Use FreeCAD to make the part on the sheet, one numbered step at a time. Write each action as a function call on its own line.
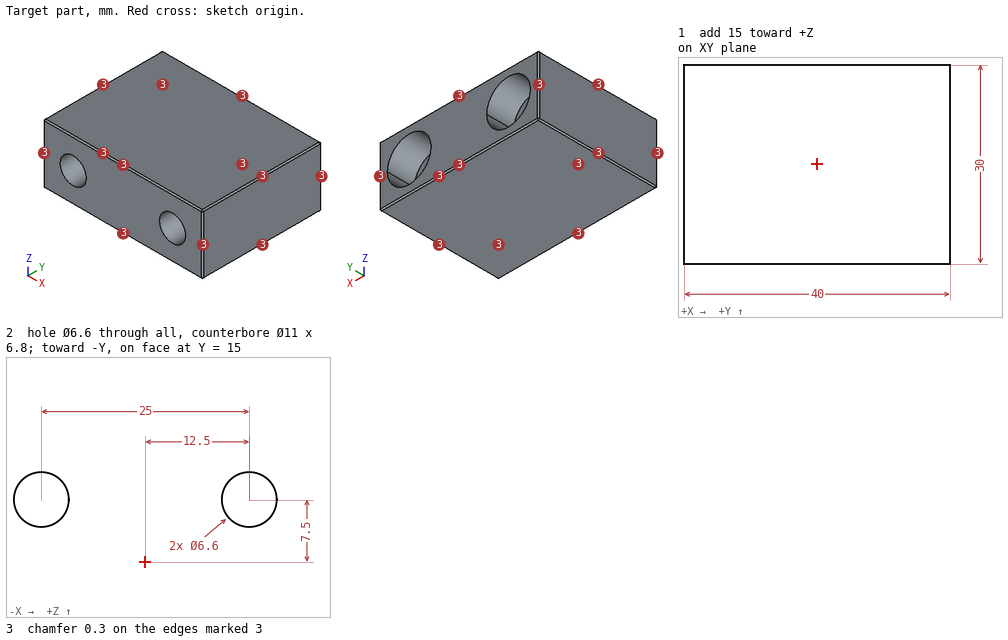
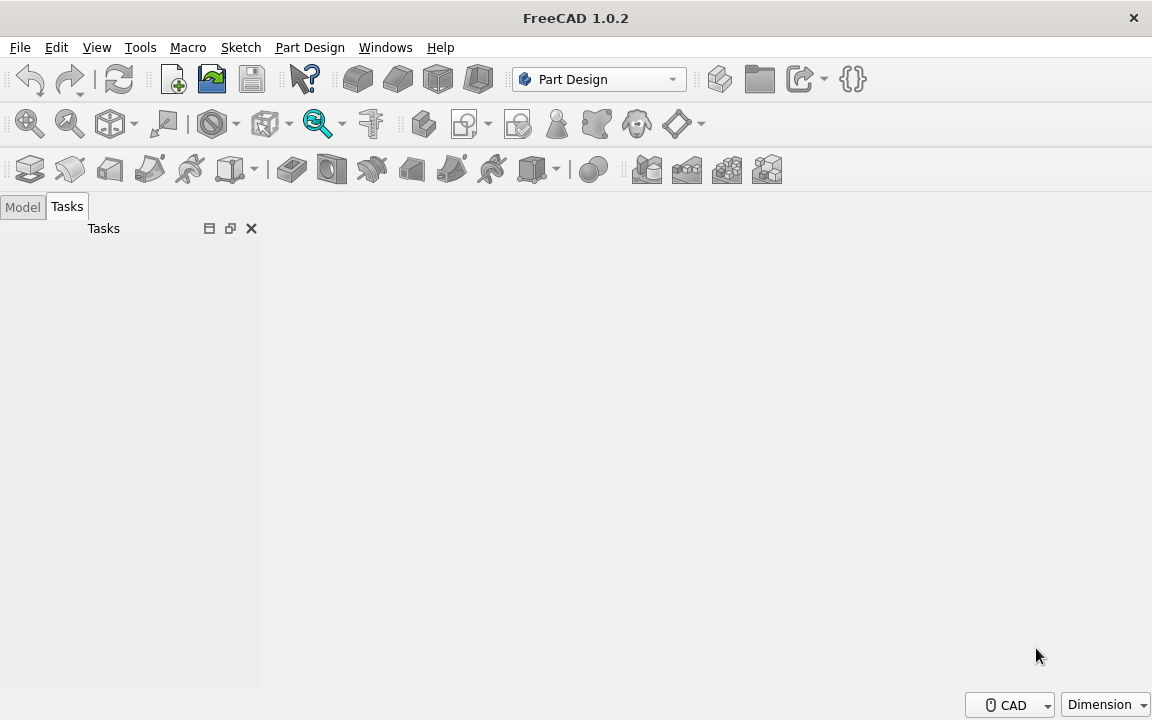
key(ctrl+n)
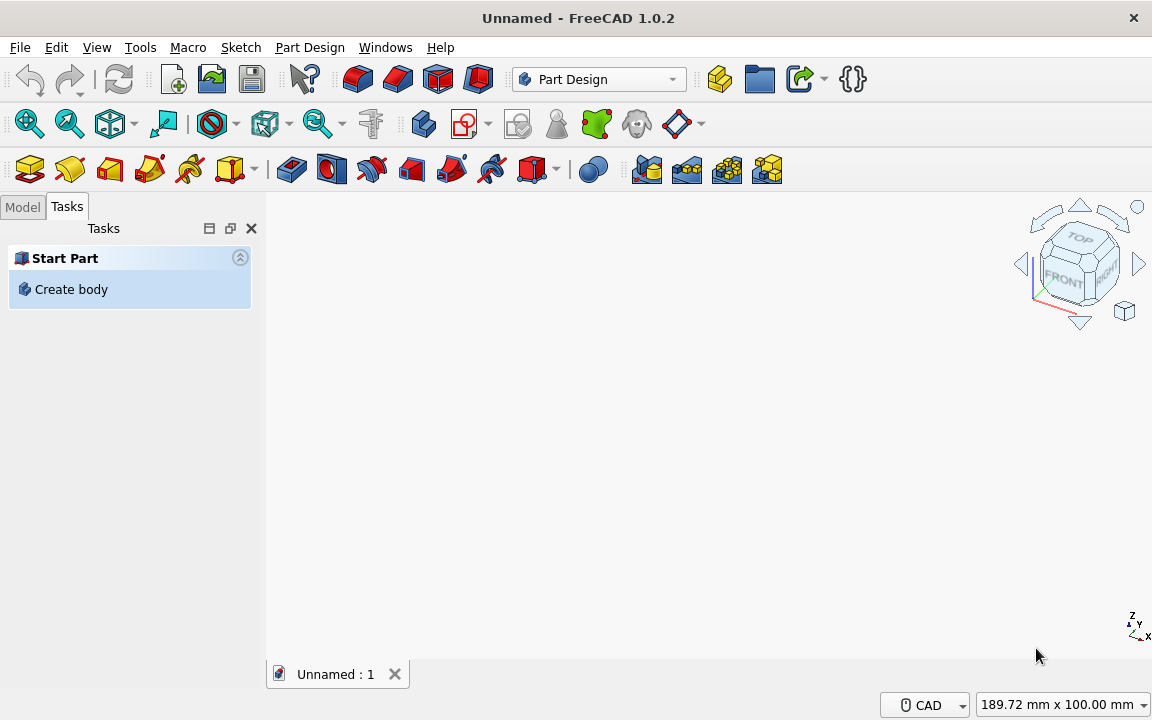
click(464, 124)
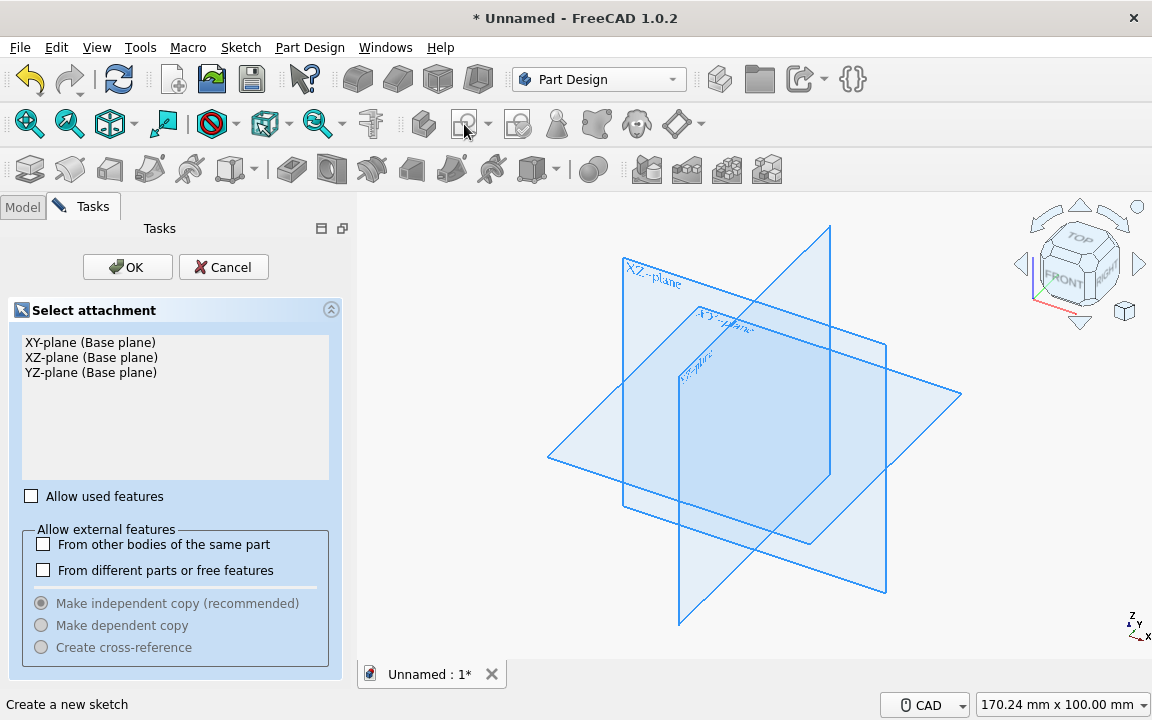
click(82, 342)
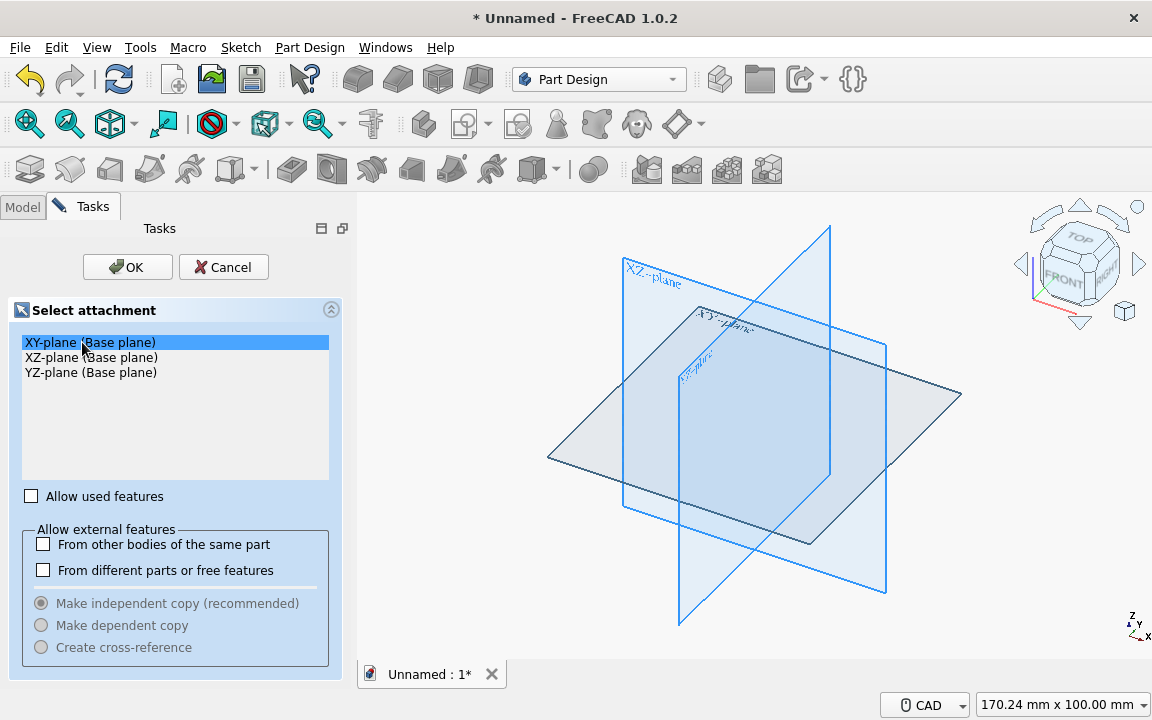
click(128, 267)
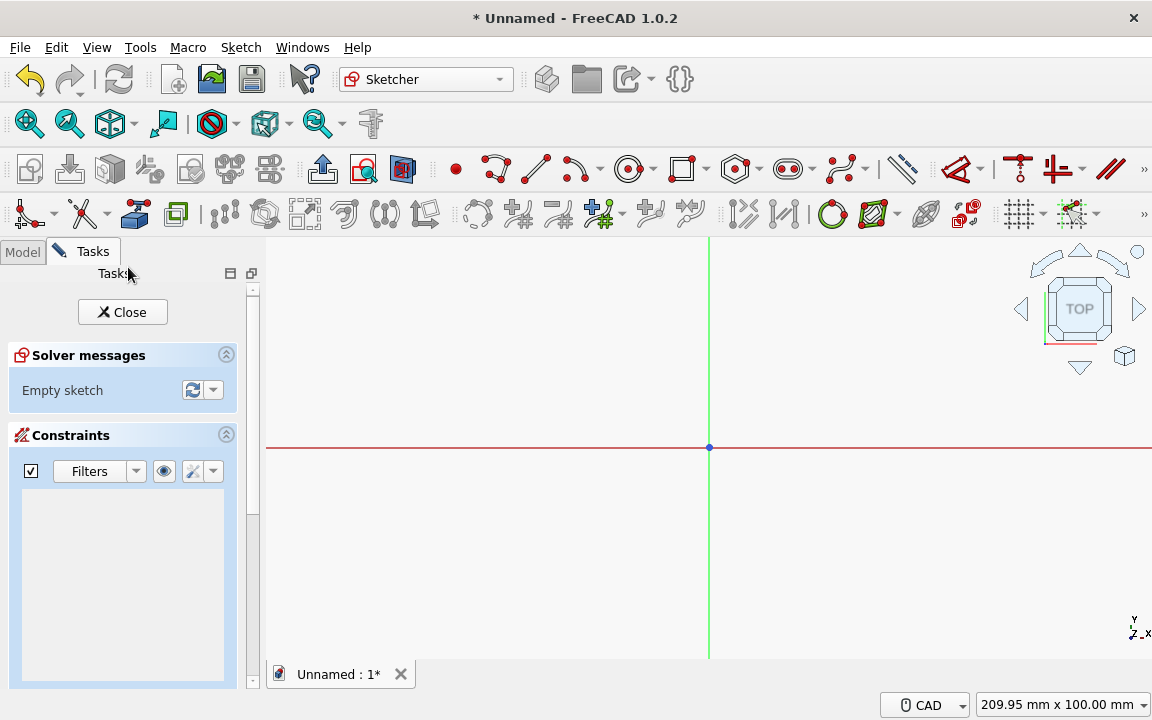
scroll(765, 448, up, 4)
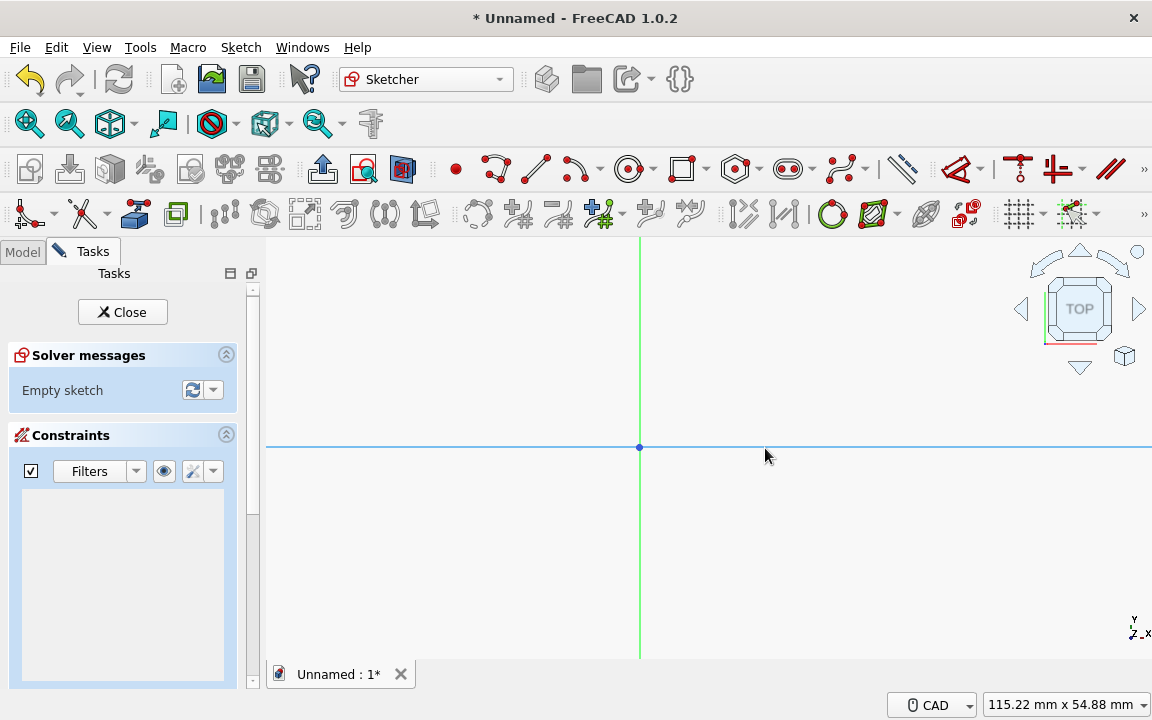
key(g)
key(v)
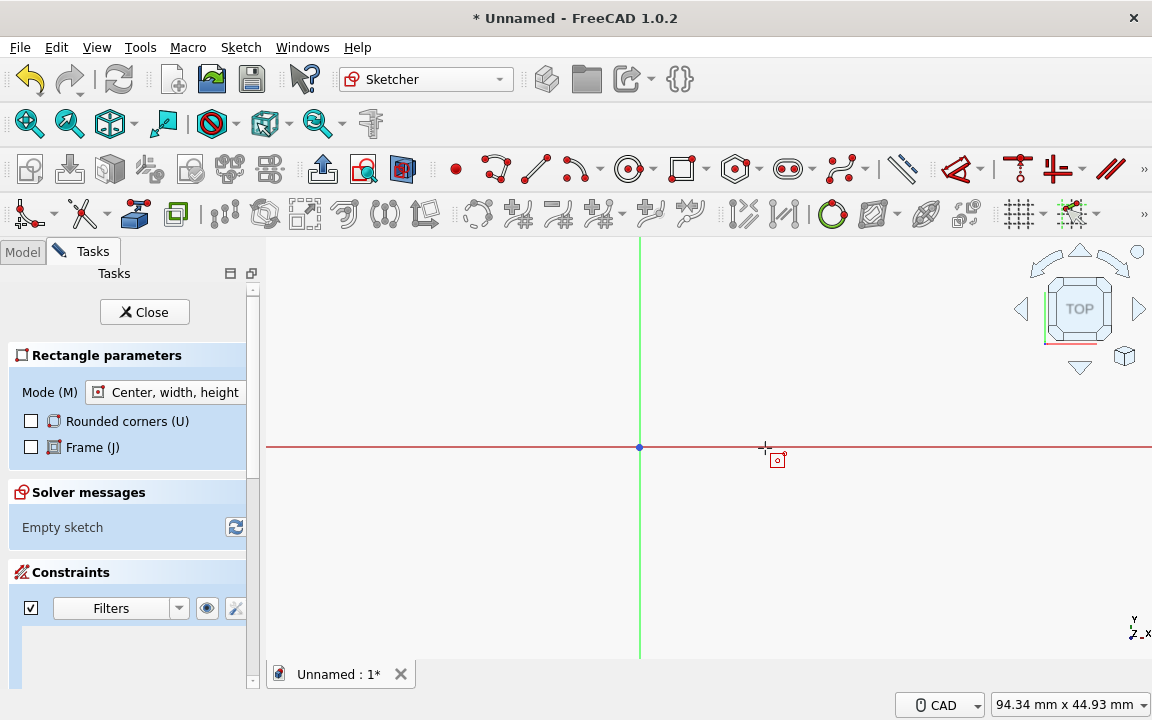
click(640, 447)
click(828, 307)
key(Escape)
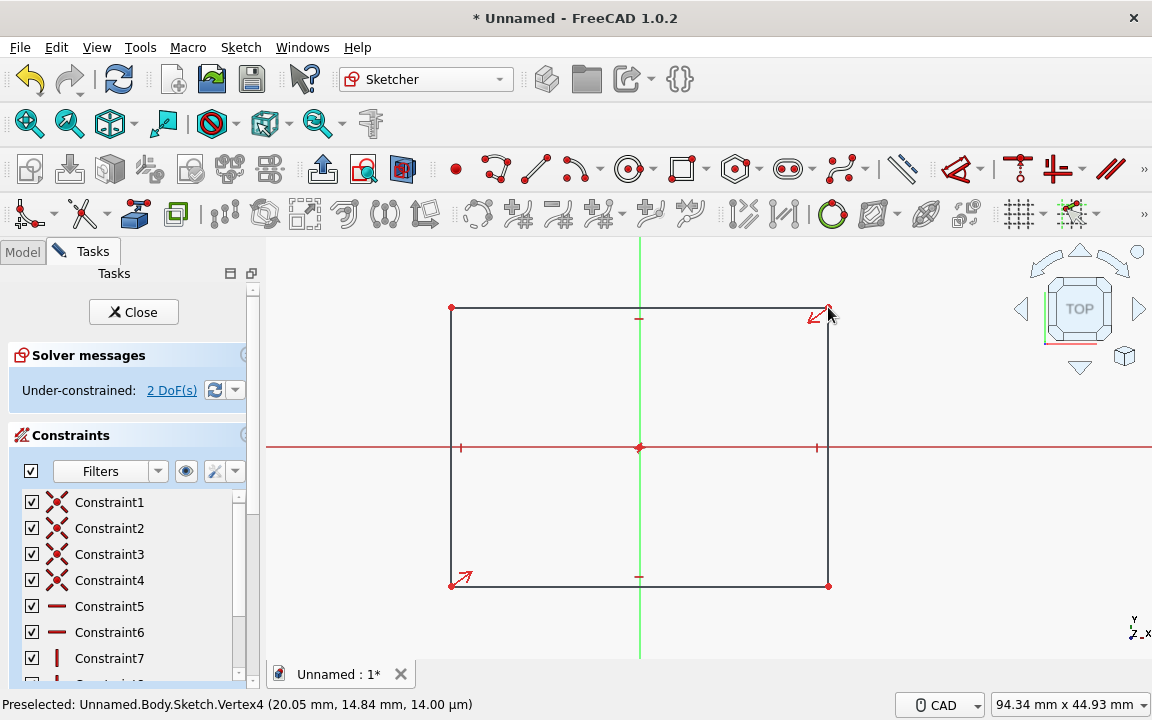
click(564, 587)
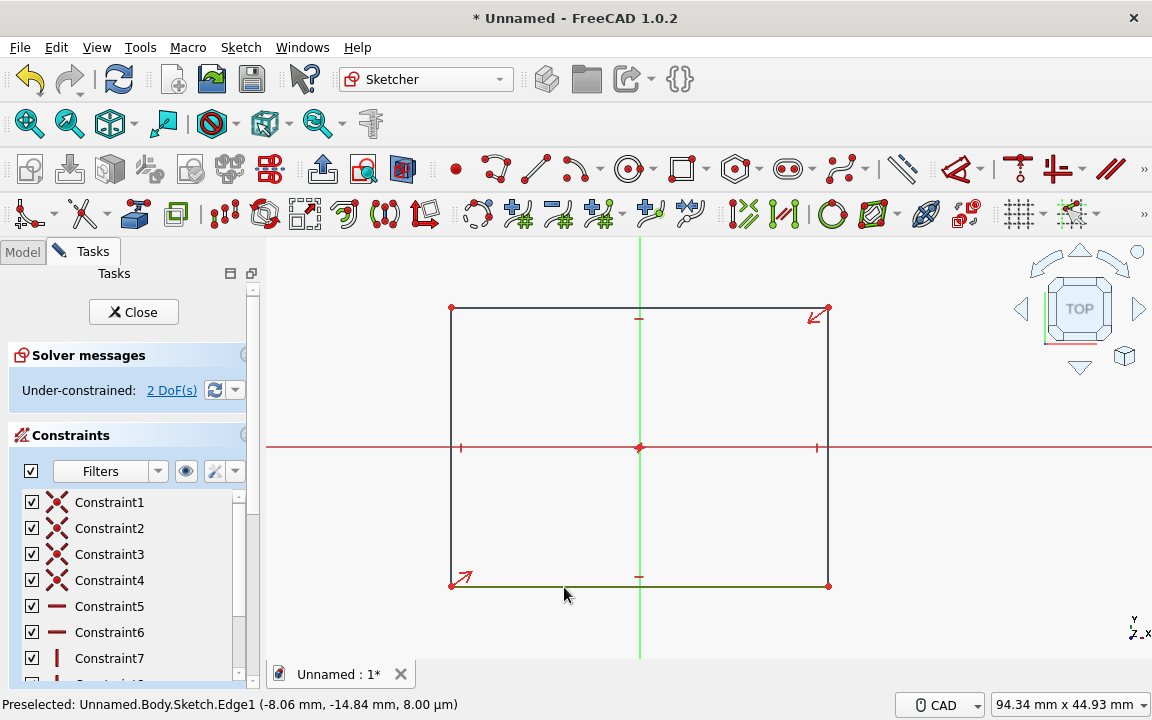
click(982, 170)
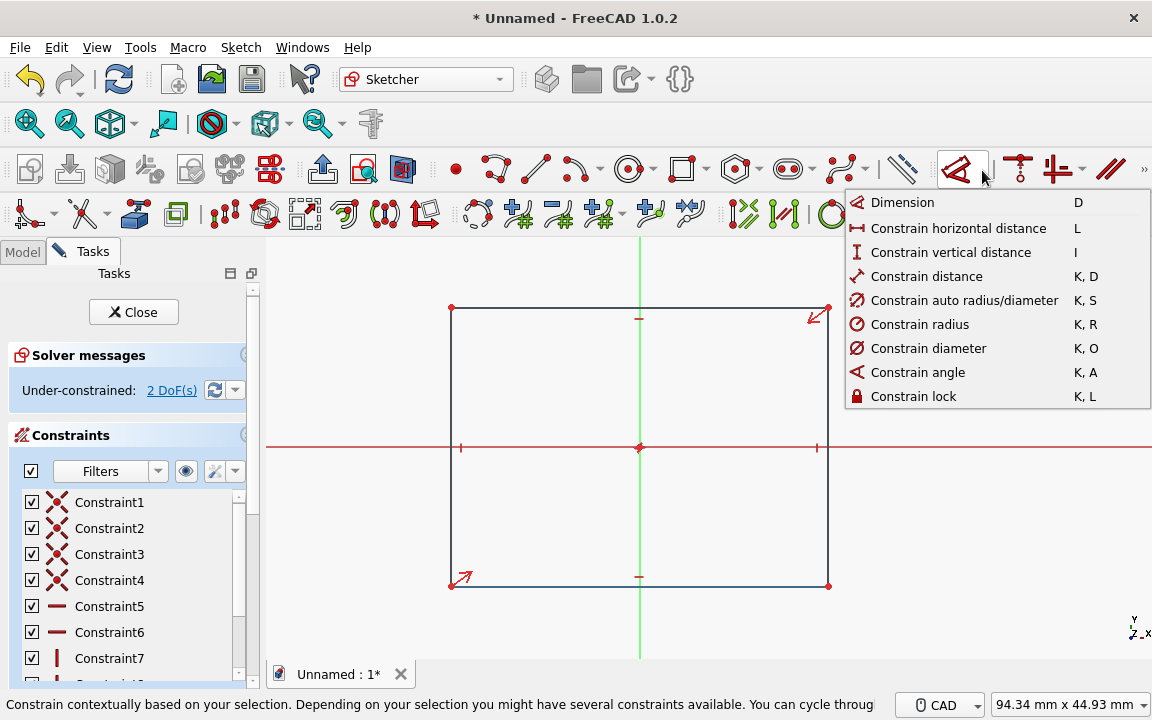
click(998, 228)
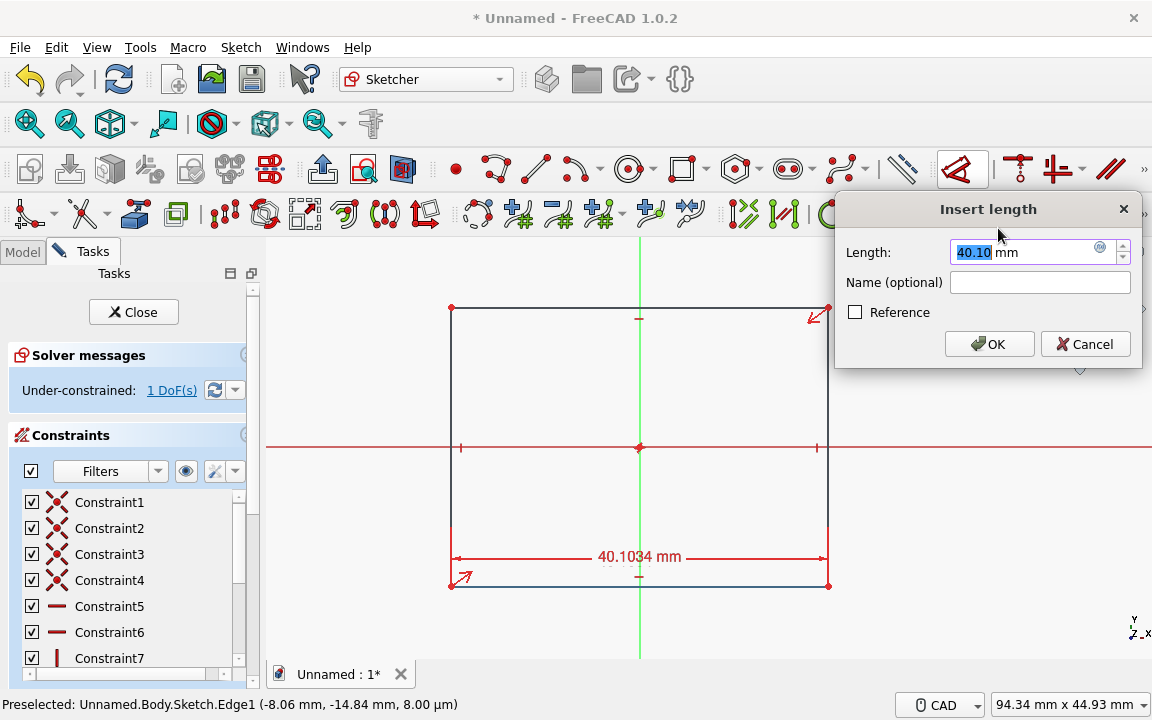
text(40)
key(Return)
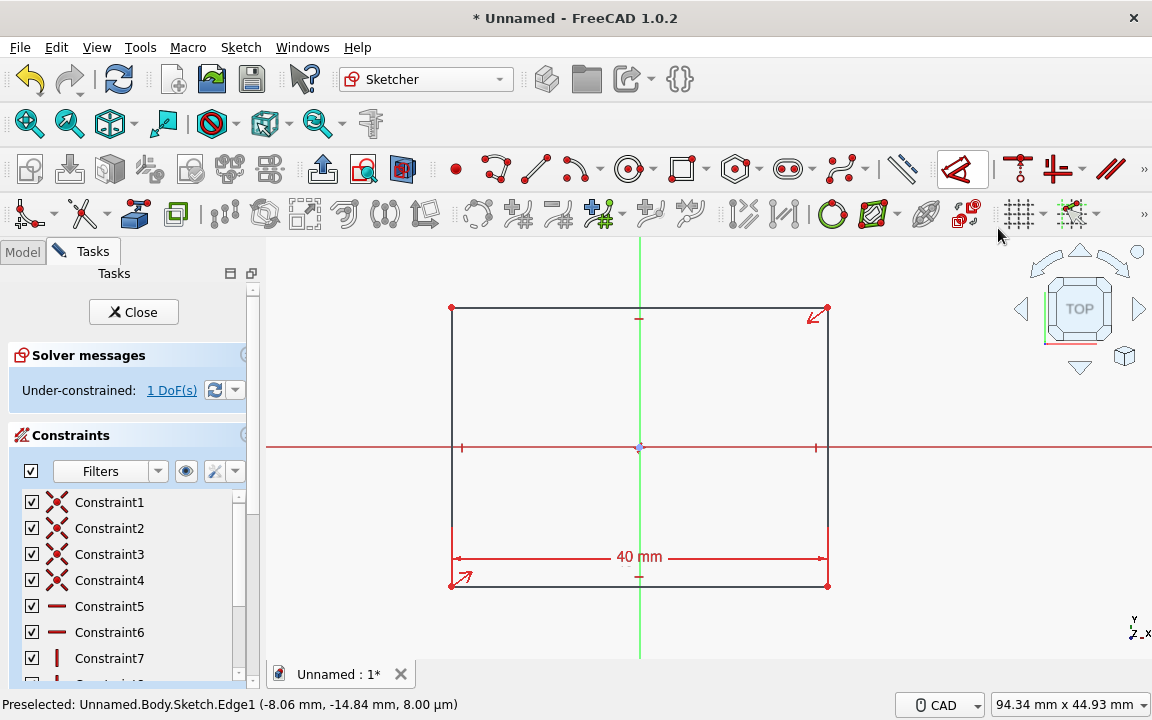
click(828, 503)